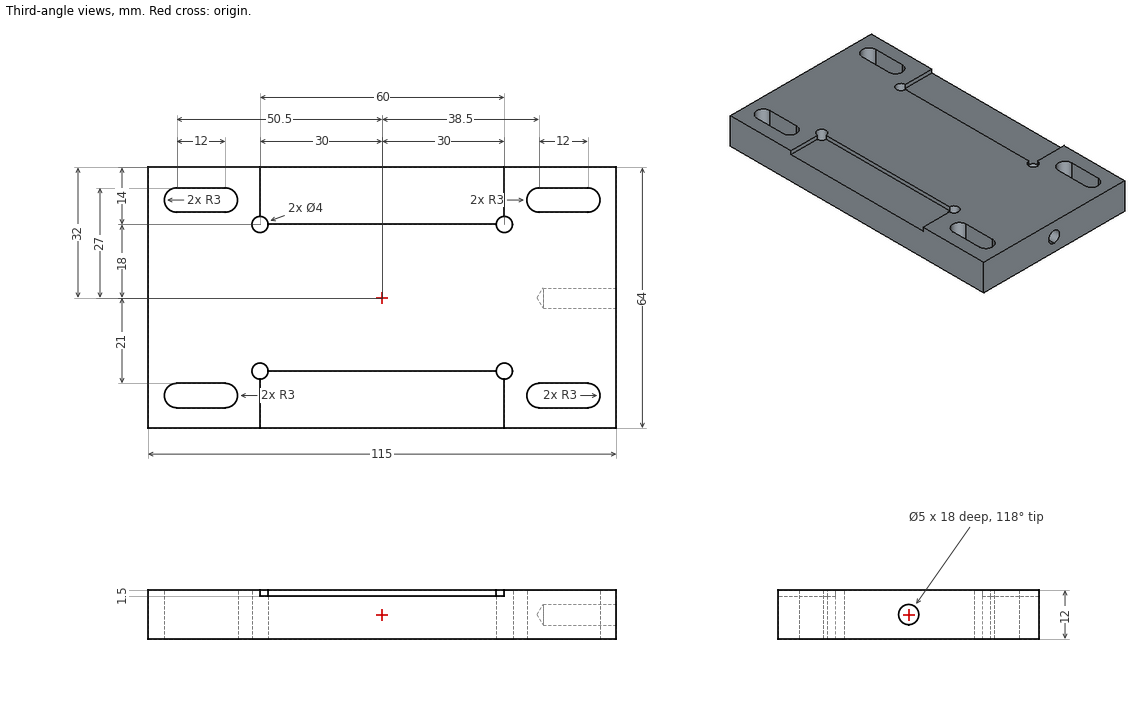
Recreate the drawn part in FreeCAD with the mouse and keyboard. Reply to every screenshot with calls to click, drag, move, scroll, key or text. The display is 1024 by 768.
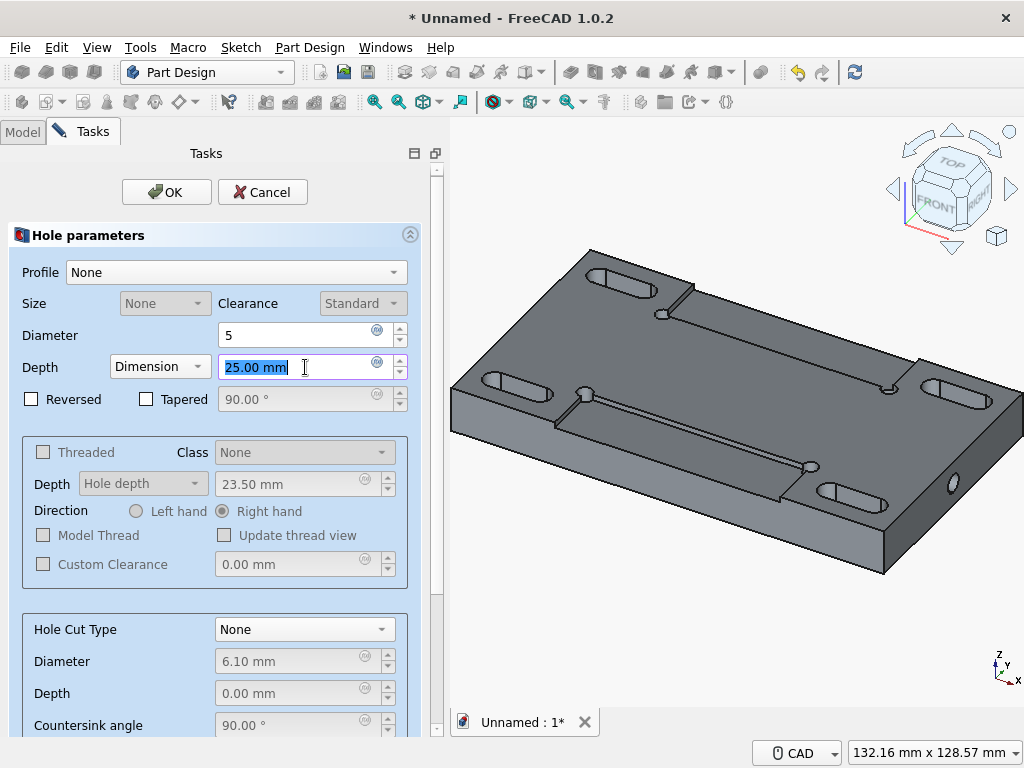
text(18)
key(Tab)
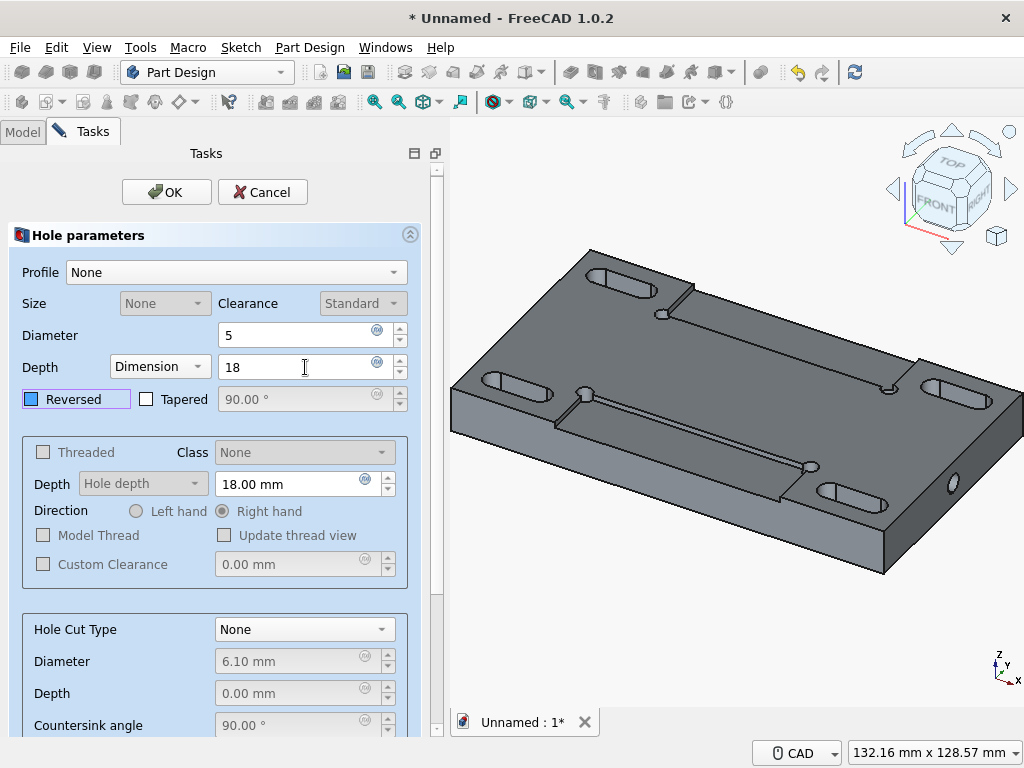
click(167, 192)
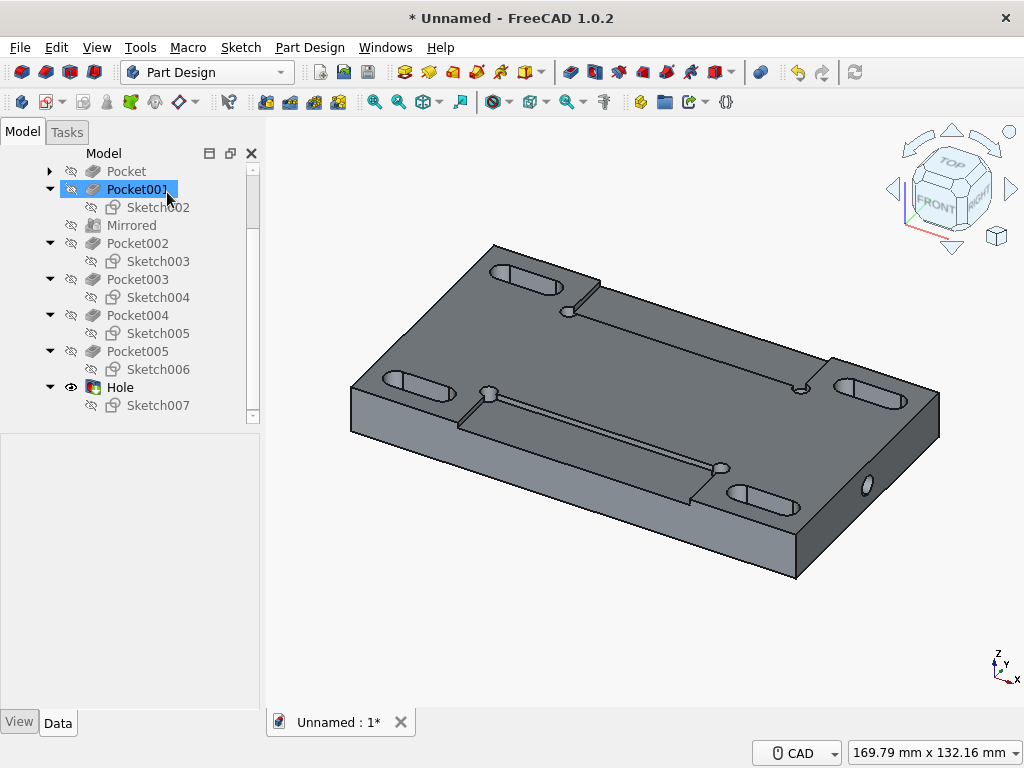
key(0)